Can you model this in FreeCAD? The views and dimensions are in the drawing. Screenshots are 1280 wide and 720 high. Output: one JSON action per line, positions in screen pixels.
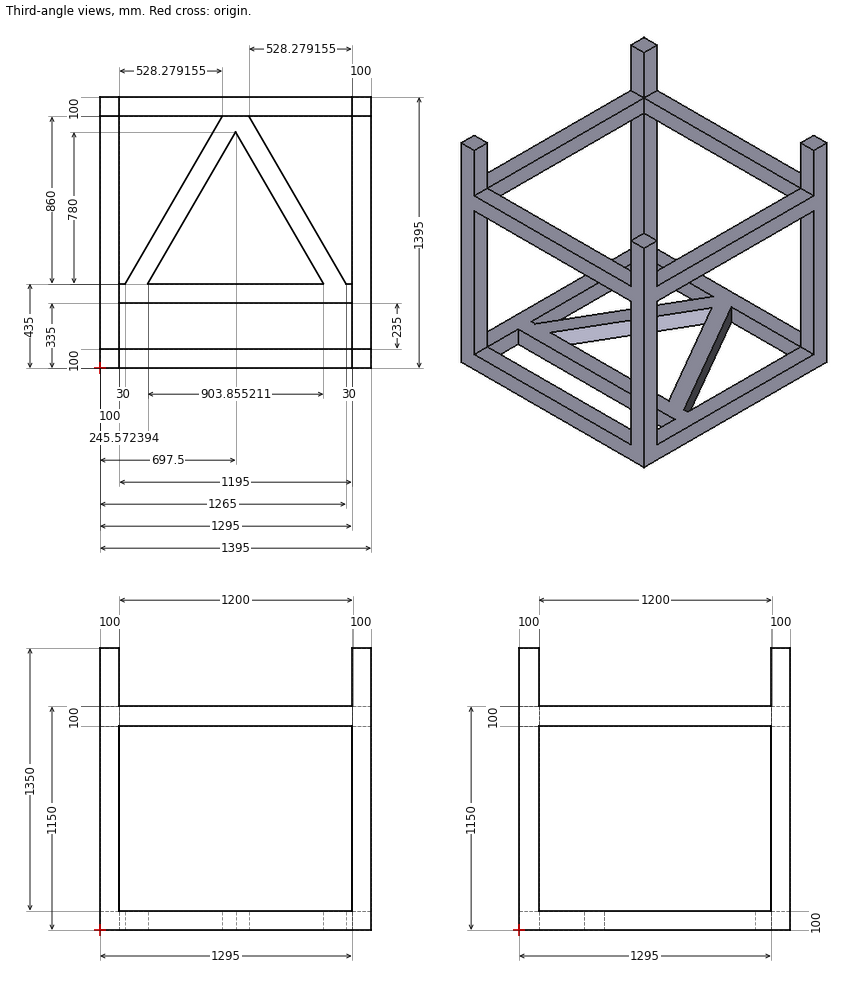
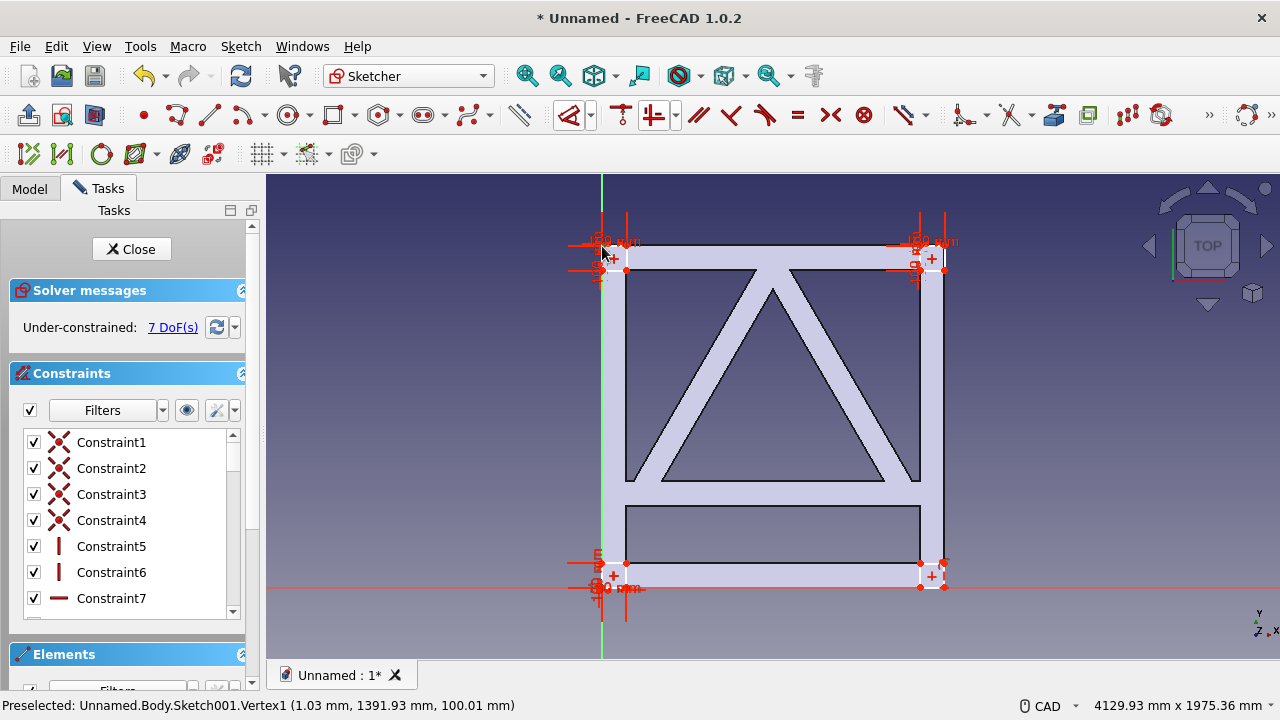
{"action": "left_click", "coordinate": [602, 508]}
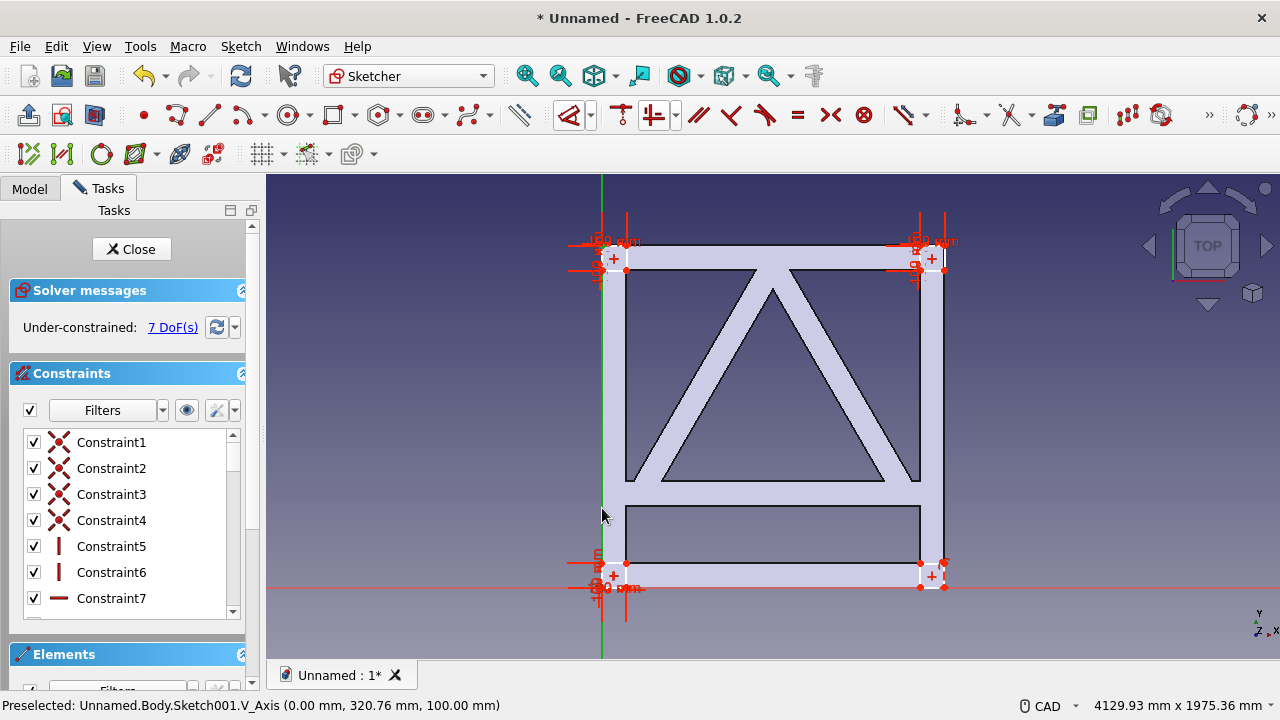
{"action": "left_click", "coordinate": [621, 116]}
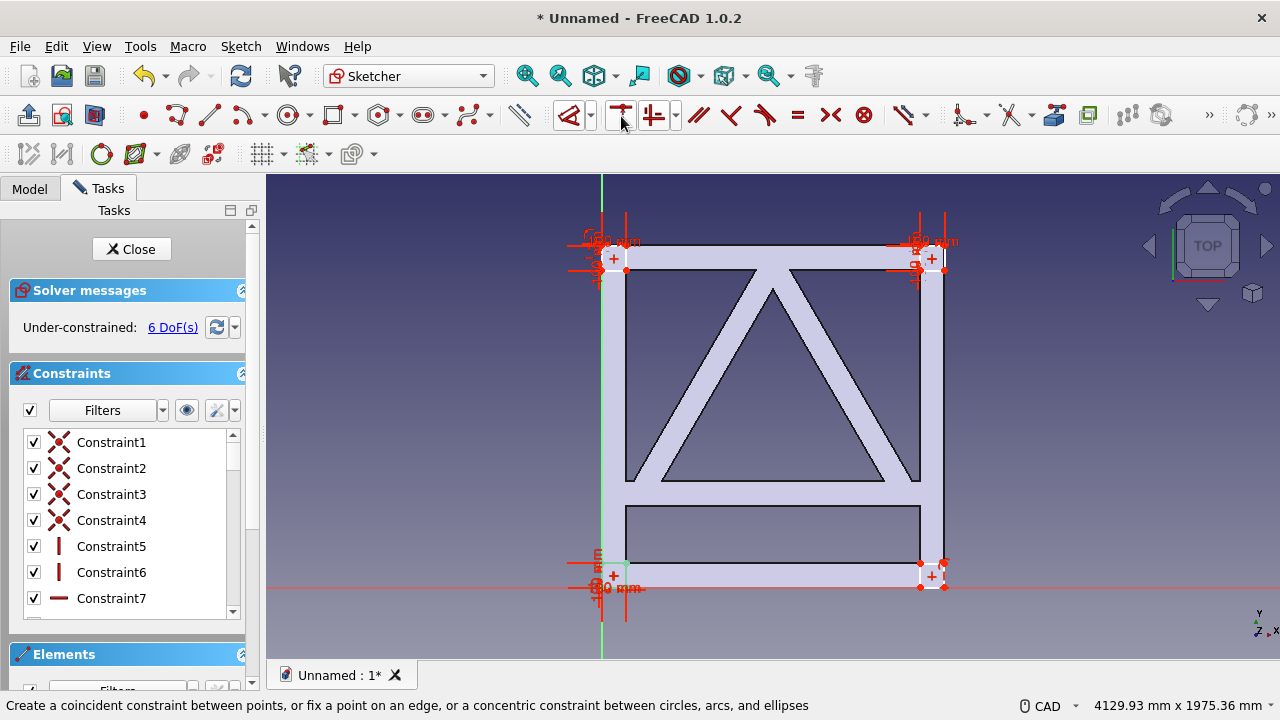
{"action": "scroll", "coordinate": [920, 574], "scroll_direction": "up", "scroll_amount": 3}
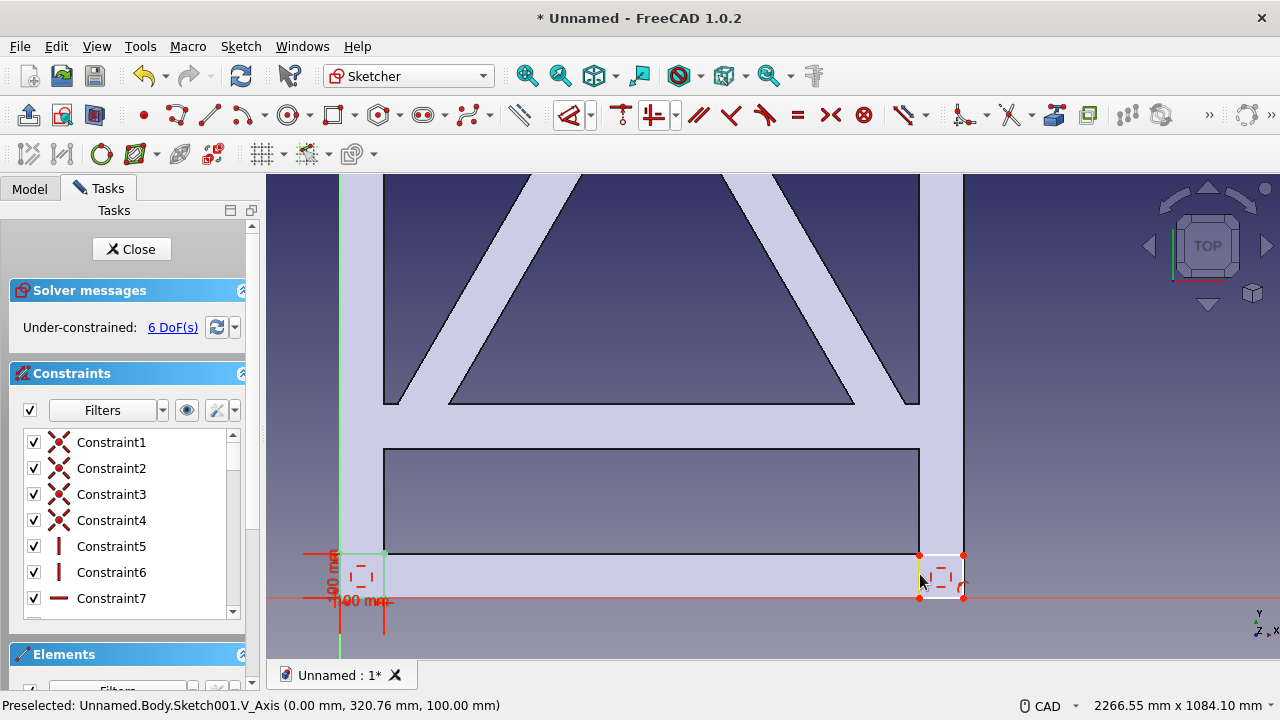
{"action": "left_click", "coordinate": [919, 572]}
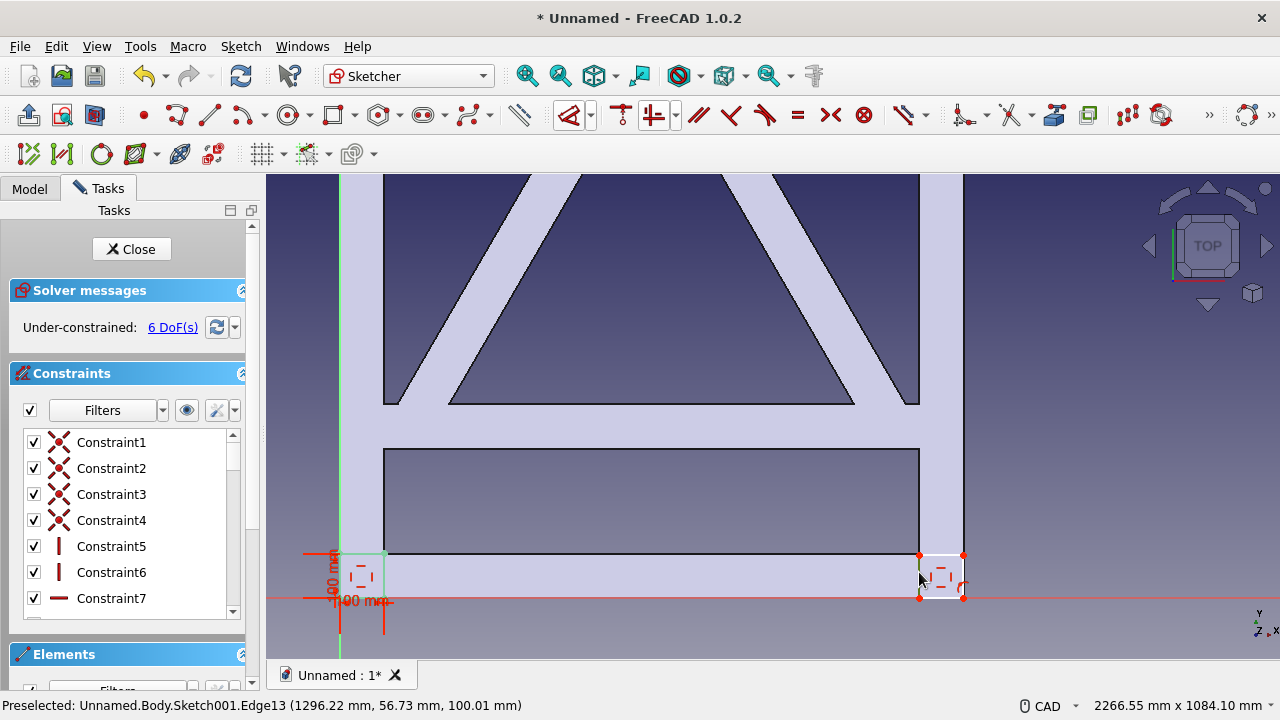
{"action": "left_click", "coordinate": [590, 116]}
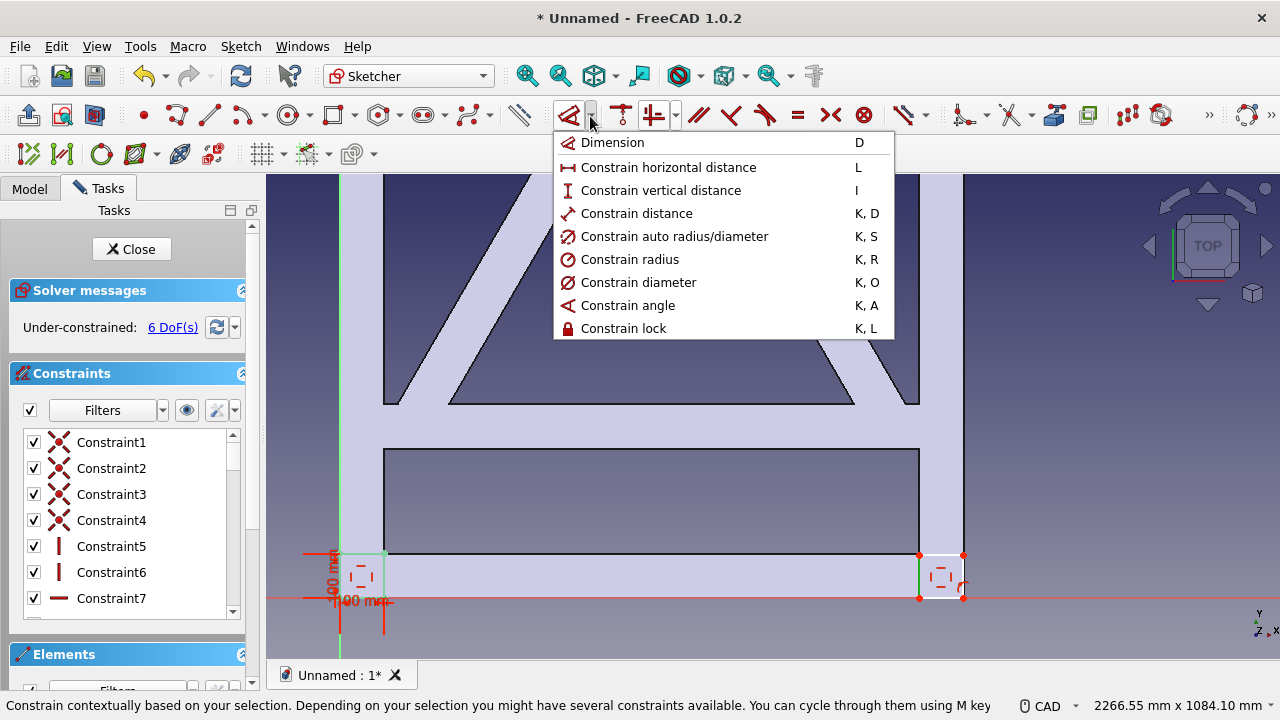
{"action": "left_click", "coordinate": [724, 190]}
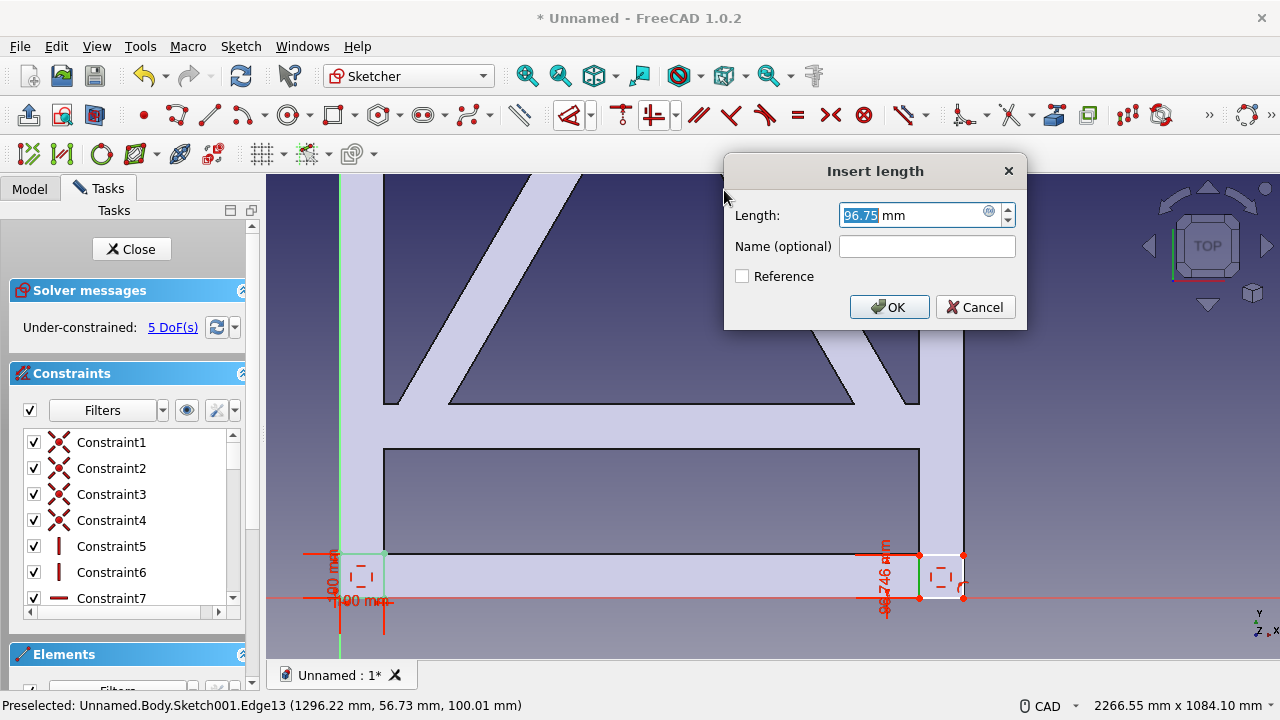
{"action": "type", "text": "100"}
{"action": "key", "text": "Return"}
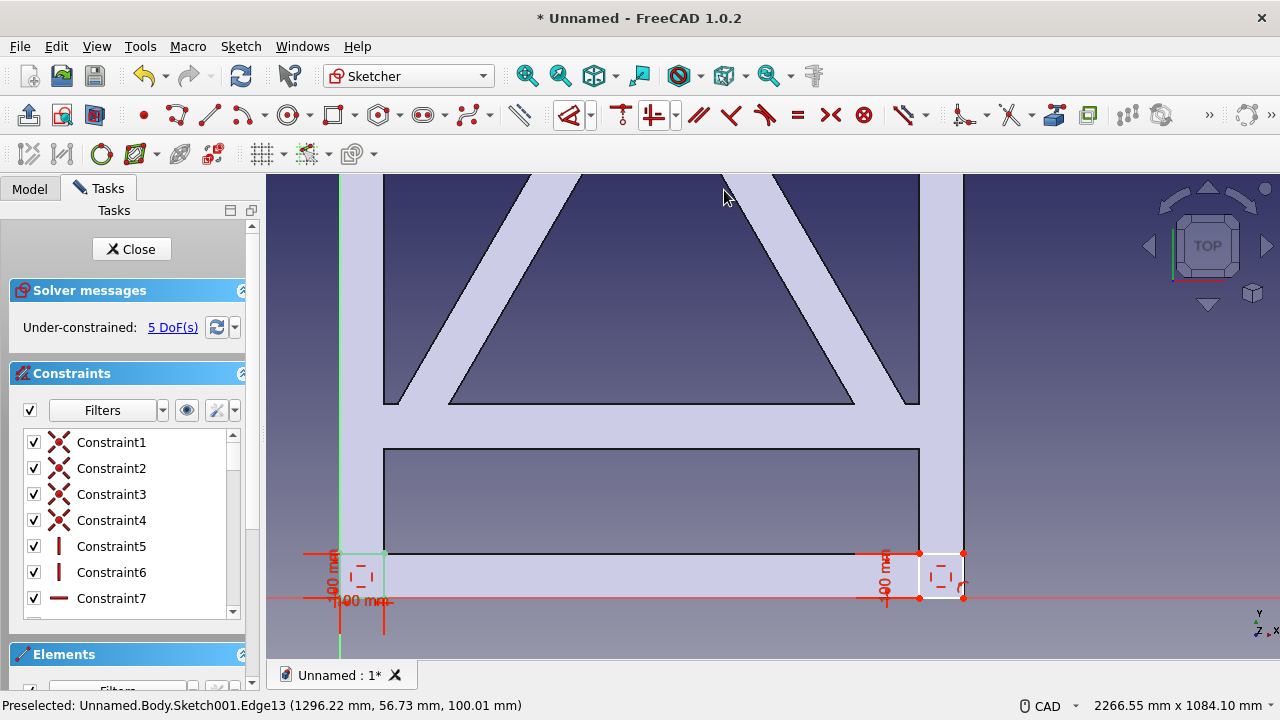
{"action": "left_click", "coordinate": [933, 598]}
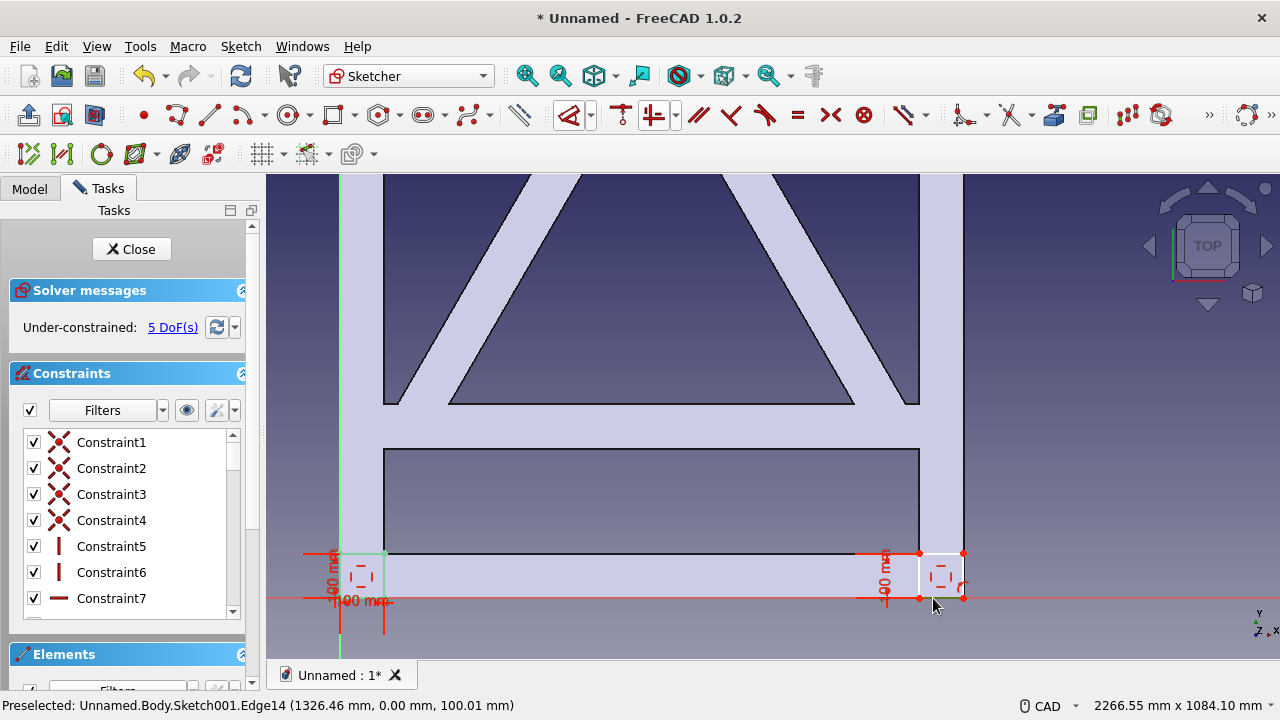
{"action": "left_click", "coordinate": [590, 116]}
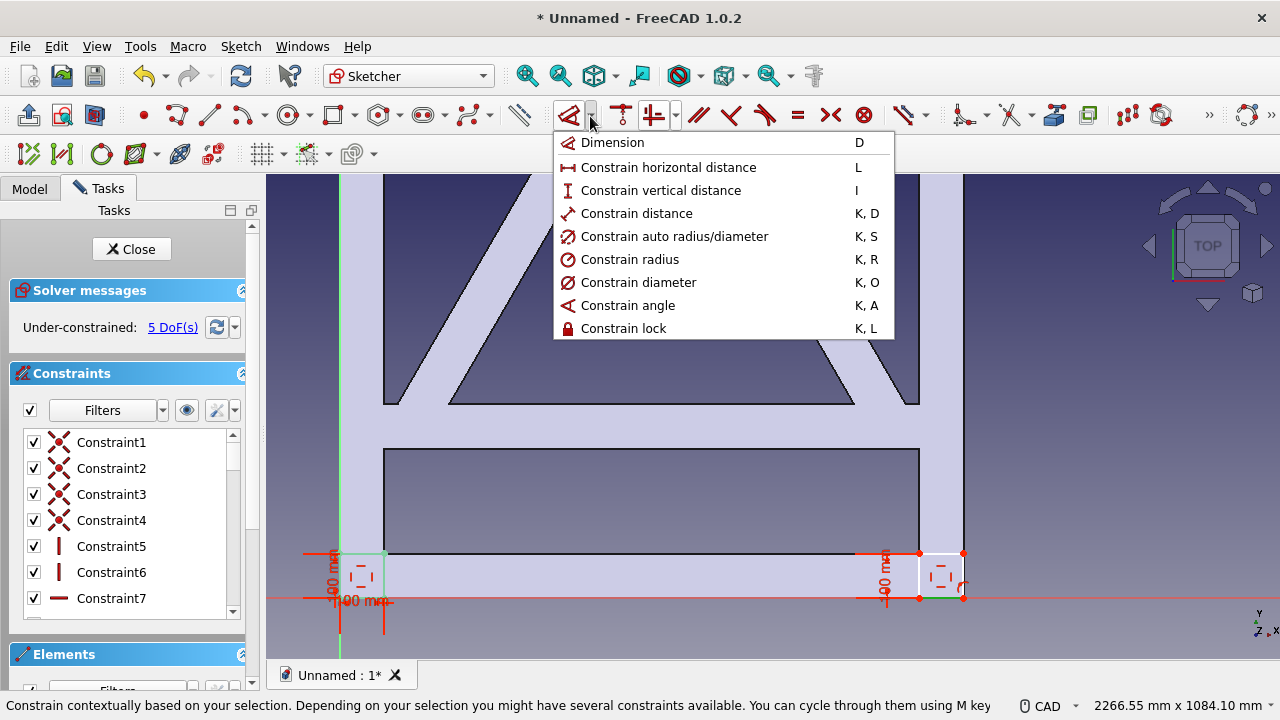
{"action": "left_click", "coordinate": [724, 168]}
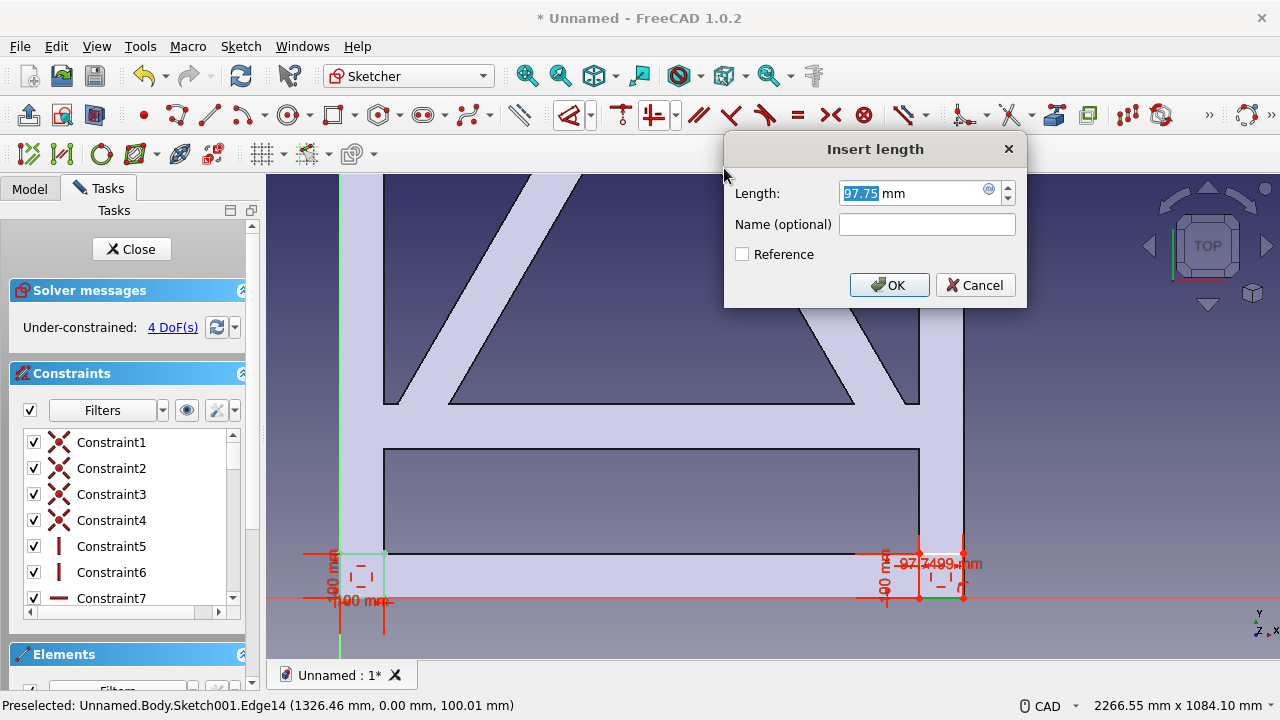
{"action": "type", "text": "100"}
{"action": "key", "text": "Return"}